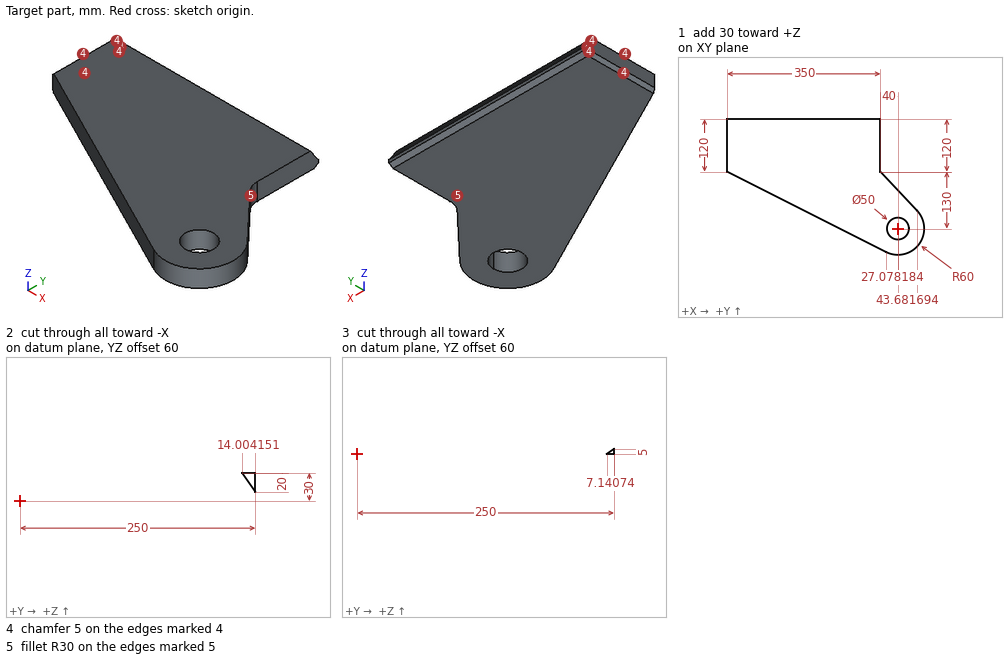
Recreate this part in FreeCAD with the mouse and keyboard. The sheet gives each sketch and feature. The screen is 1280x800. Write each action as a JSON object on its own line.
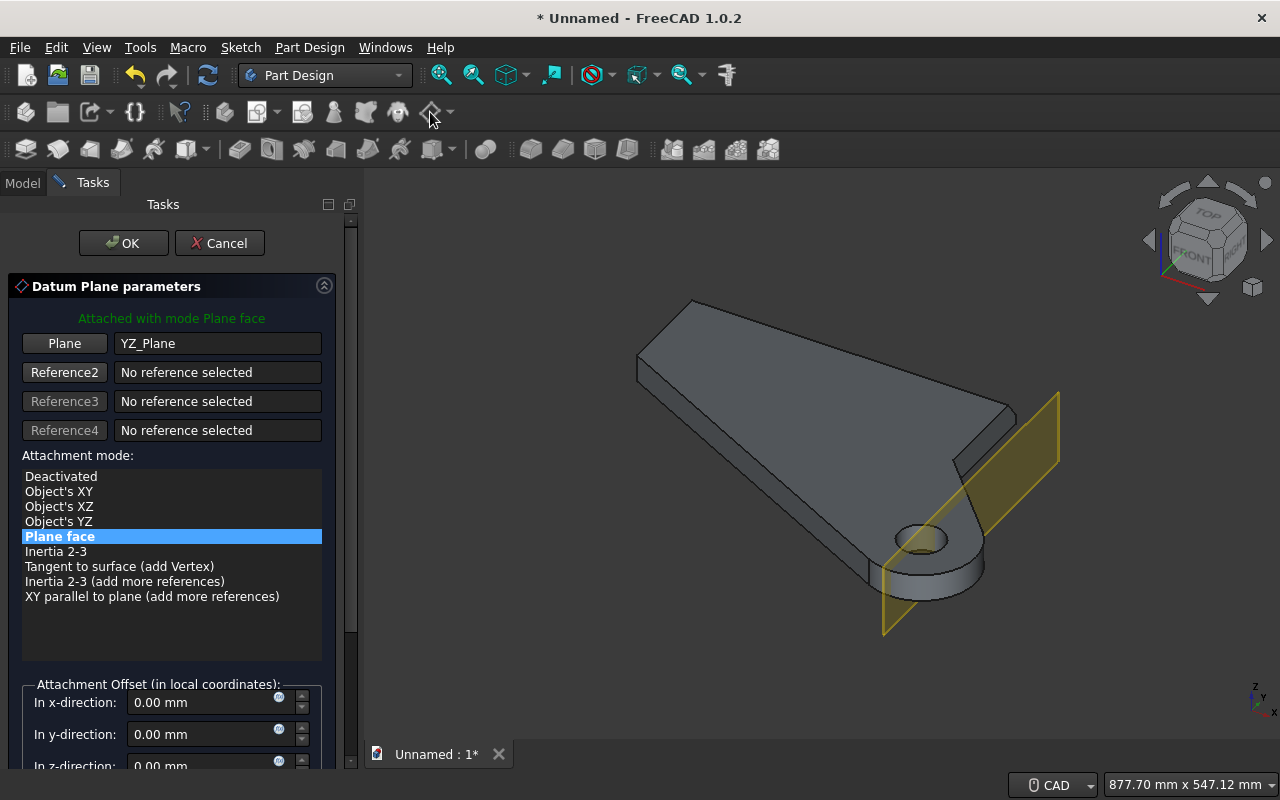
{"action": "scroll", "coordinate": [351, 491], "scroll_direction": "down", "scroll_amount": 2}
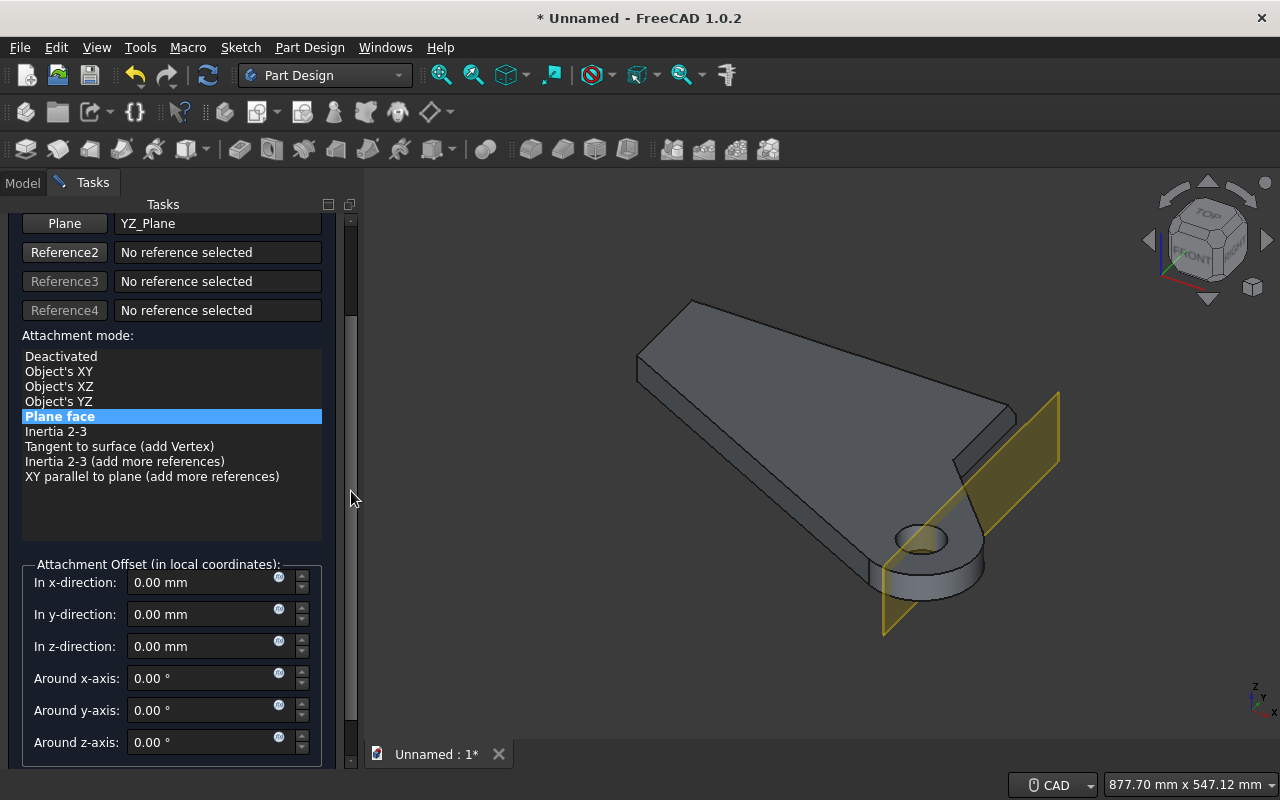
{"action": "triple_click", "coordinate": [210, 646]}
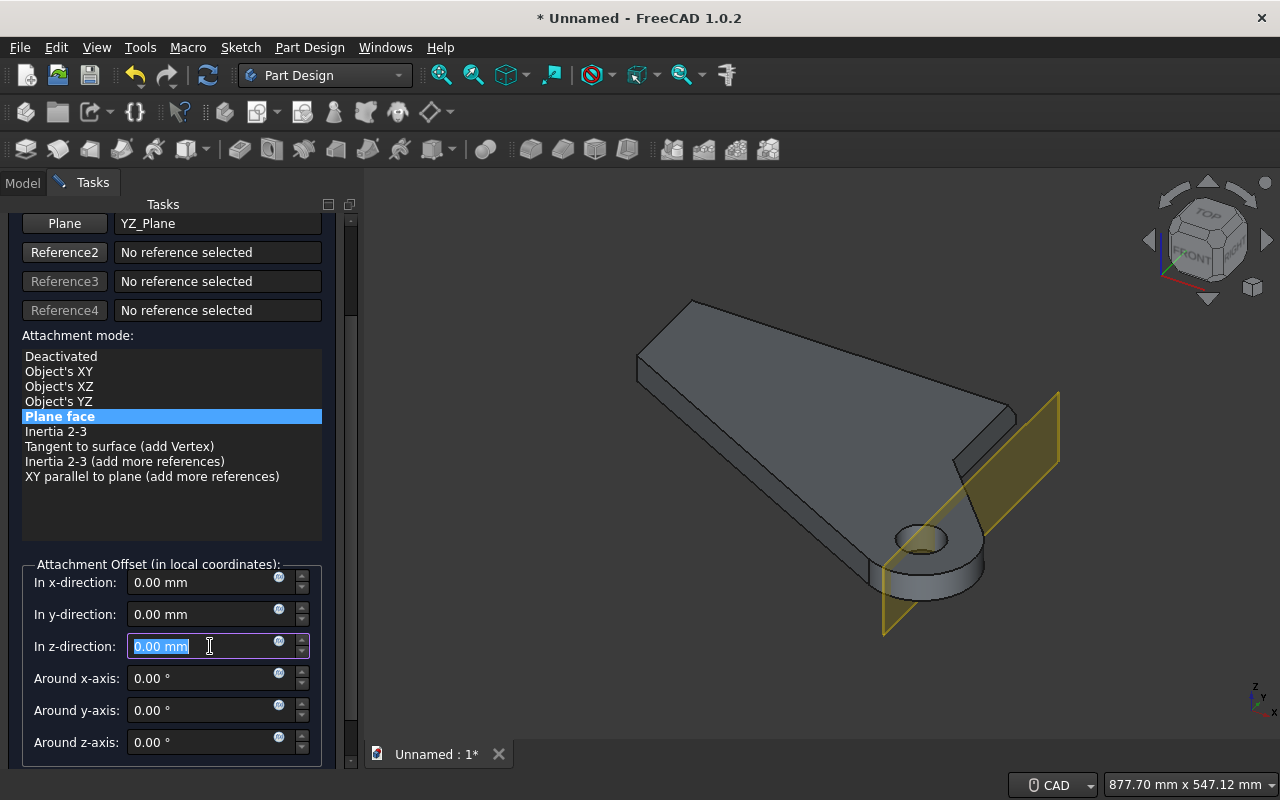
{"action": "type", "text": "60"}
{"action": "key", "text": "Tab"}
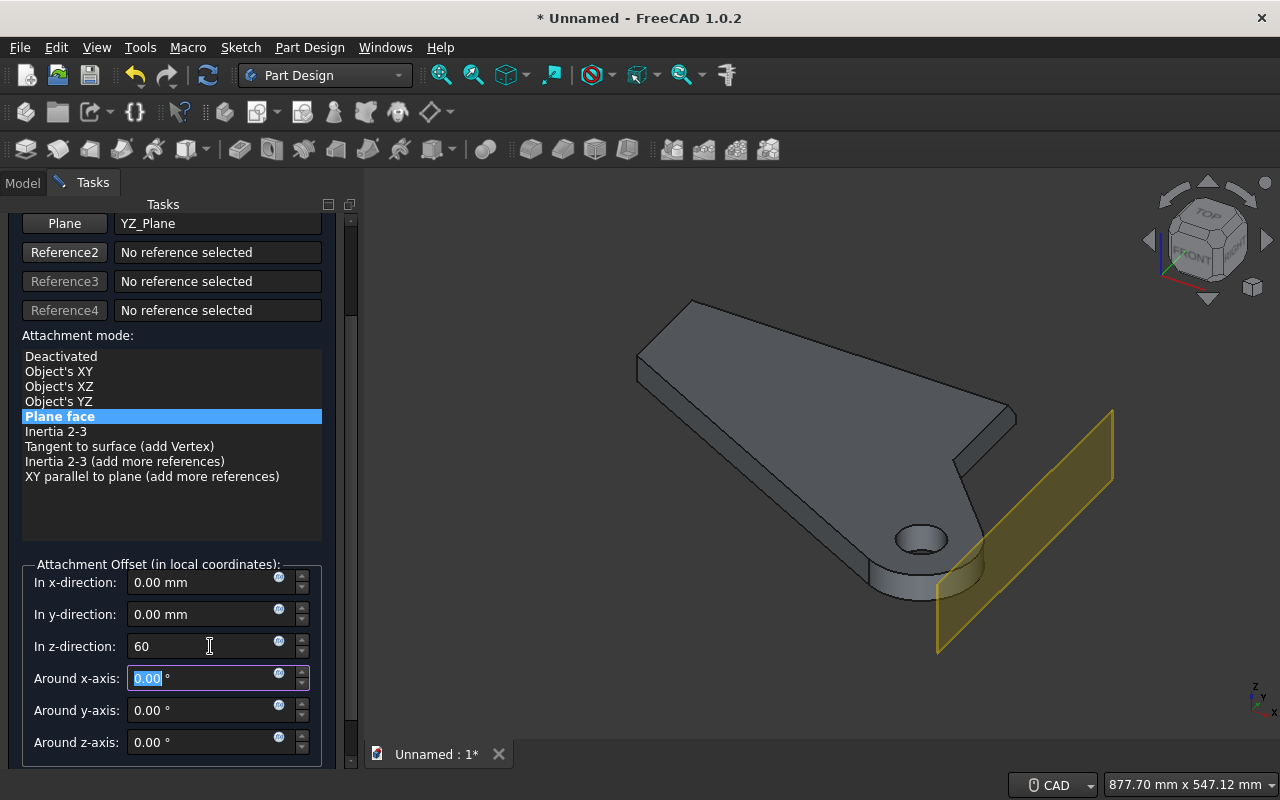
{"action": "scroll", "coordinate": [351, 491], "scroll_direction": "up", "scroll_amount": 3}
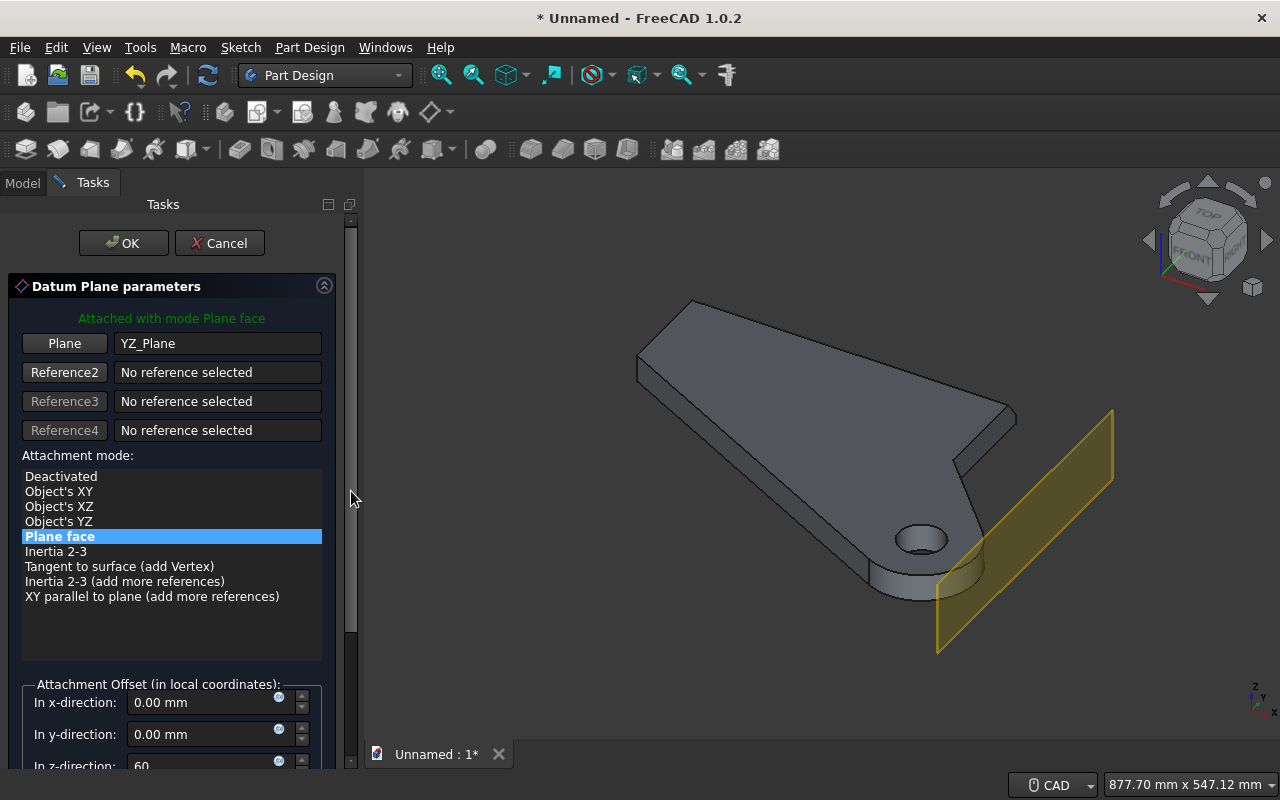
{"action": "left_click", "coordinate": [124, 243]}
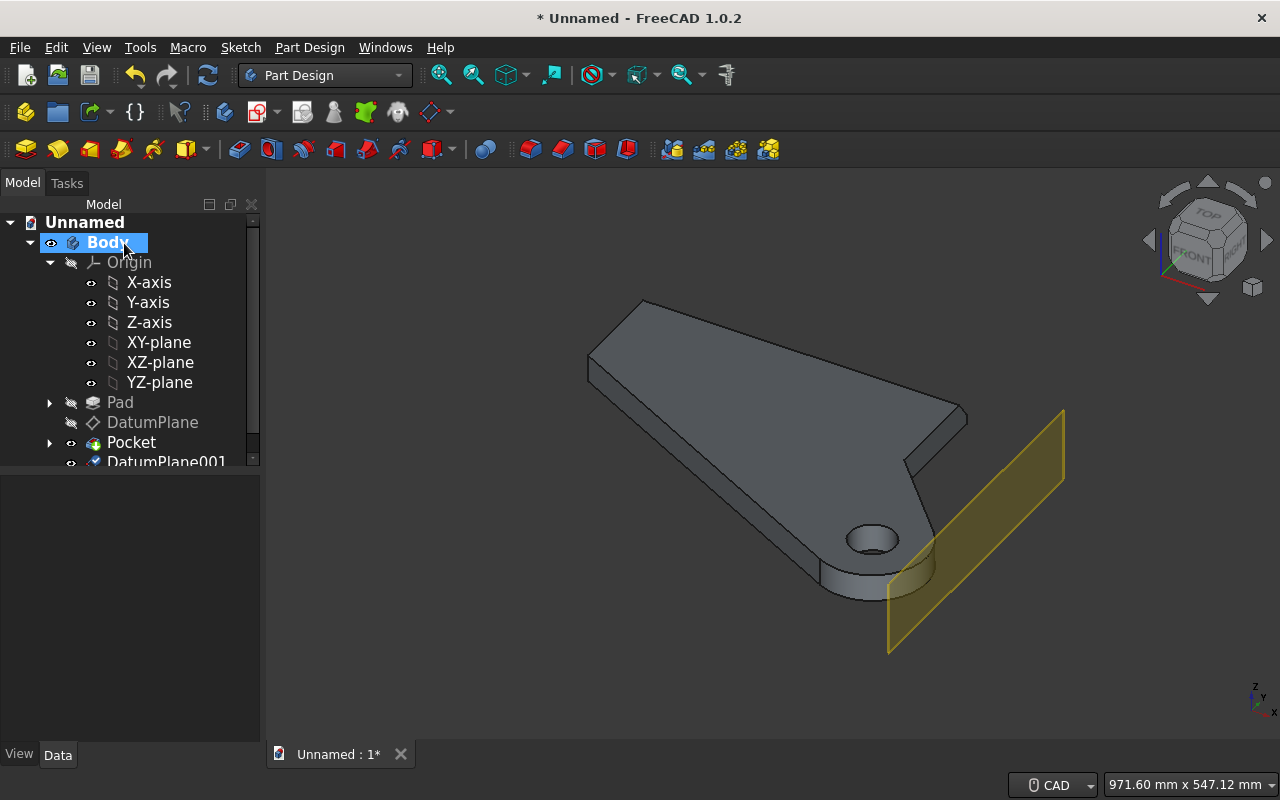
{"action": "left_click", "coordinate": [116, 463]}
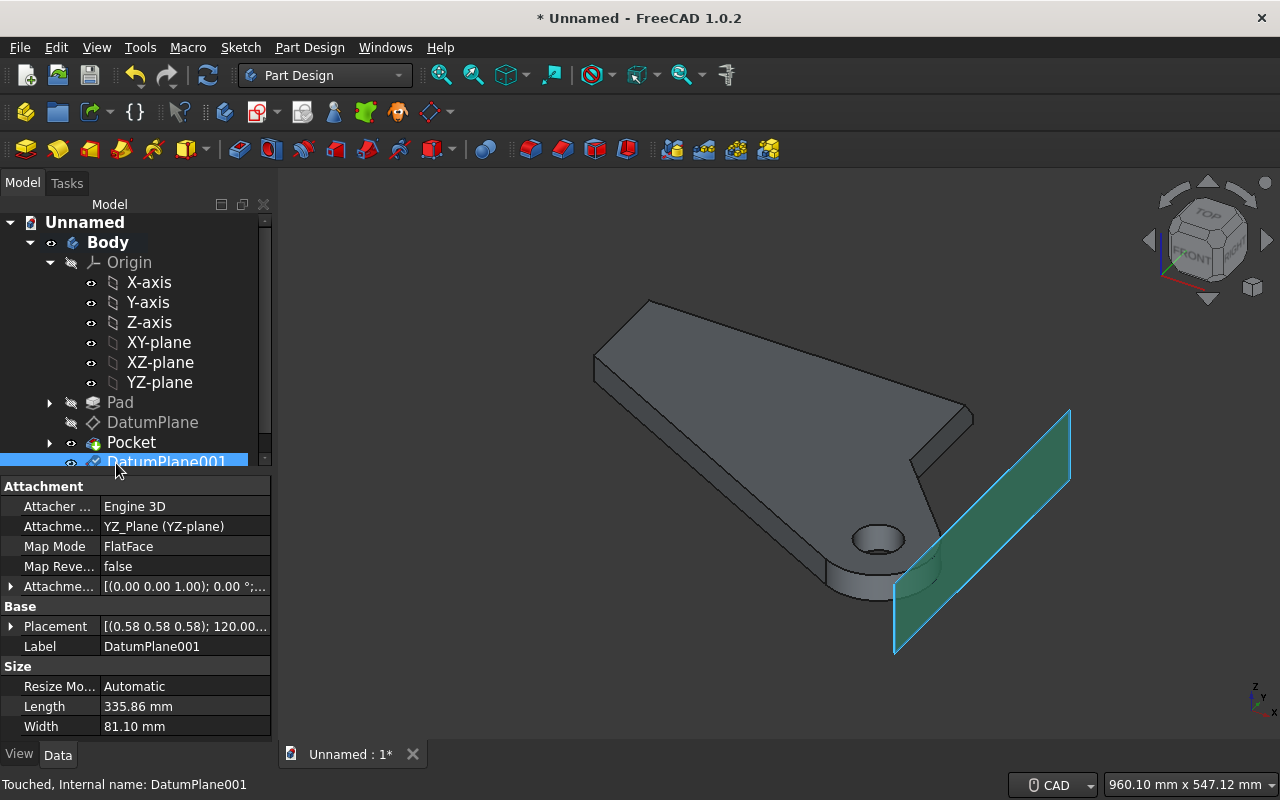
{"action": "left_click", "coordinate": [258, 112]}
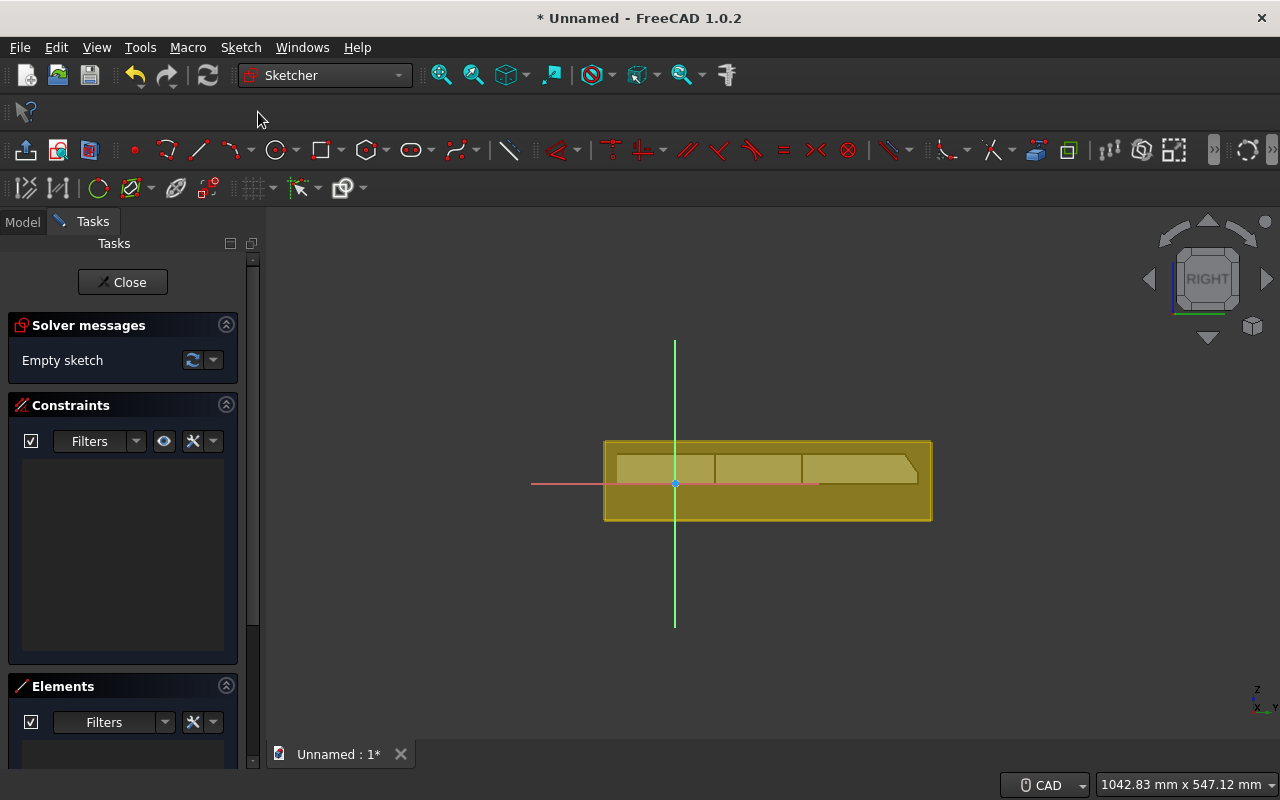
{"action": "scroll", "coordinate": [926, 482], "scroll_direction": "up", "scroll_amount": 15}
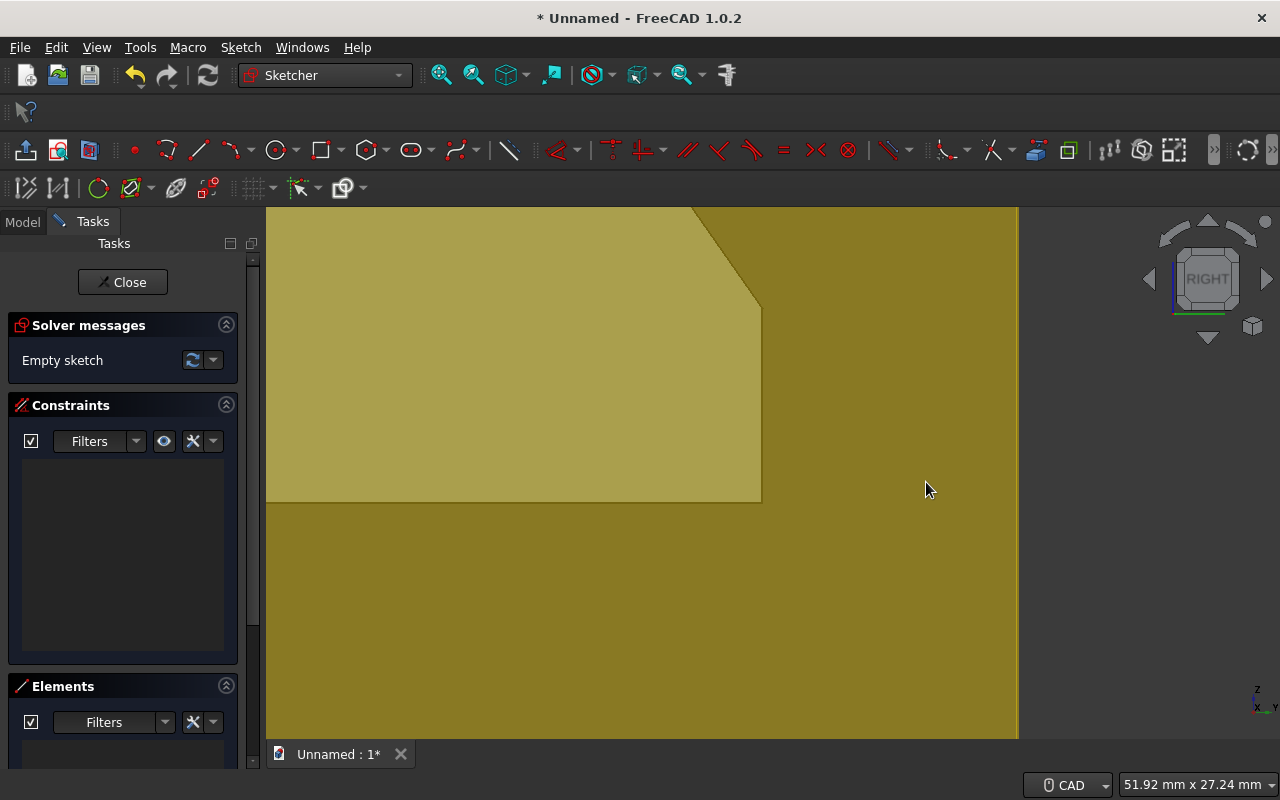
{"action": "scroll", "coordinate": [688, 447], "scroll_direction": "up", "scroll_amount": 6}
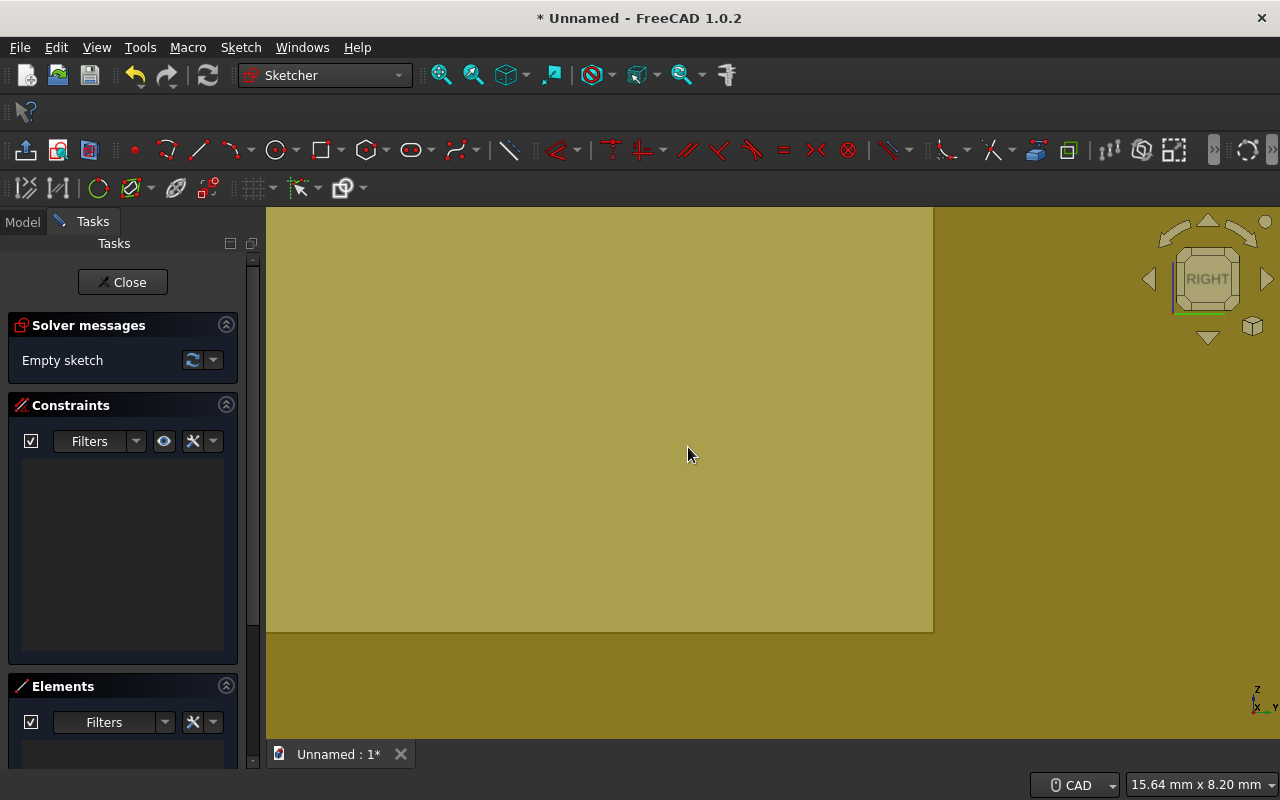
{"action": "left_click", "coordinate": [168, 150]}